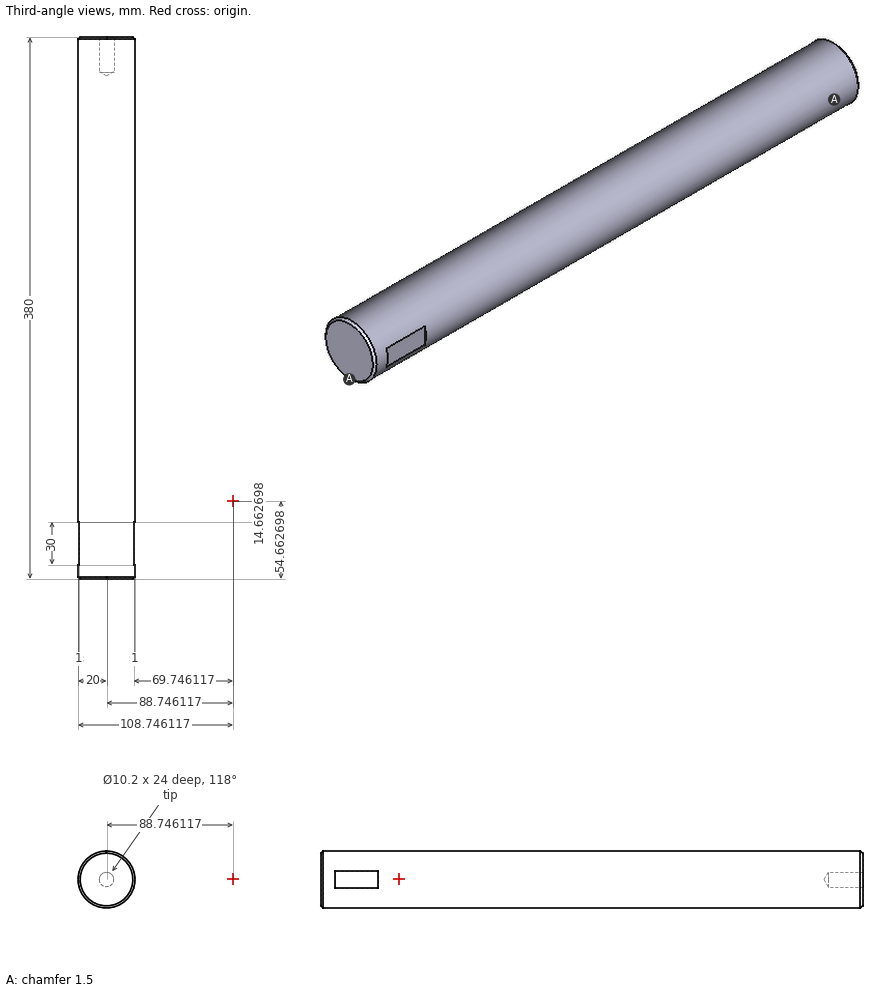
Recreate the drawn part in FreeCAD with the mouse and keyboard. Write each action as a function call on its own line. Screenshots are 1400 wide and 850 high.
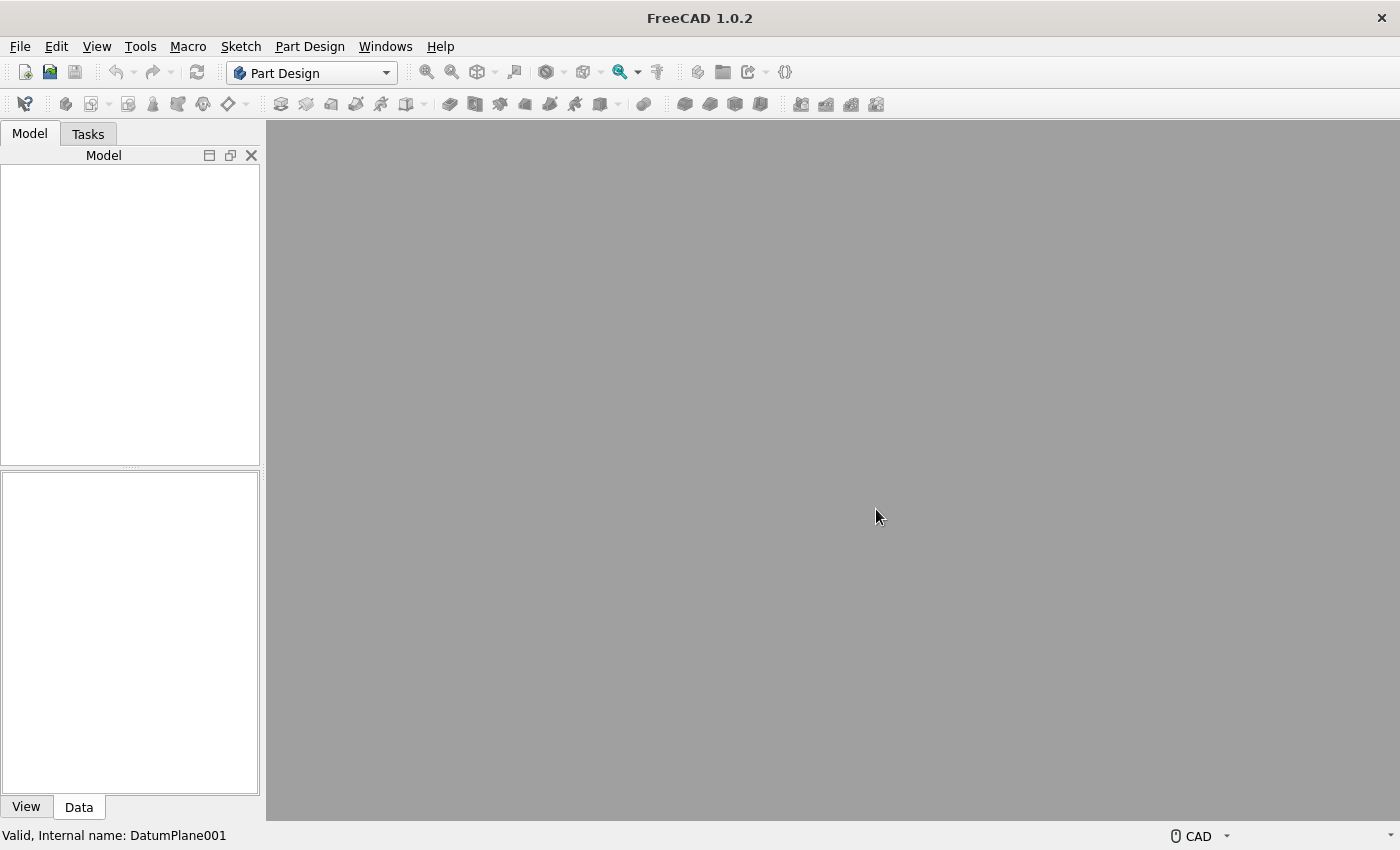
click(25, 72)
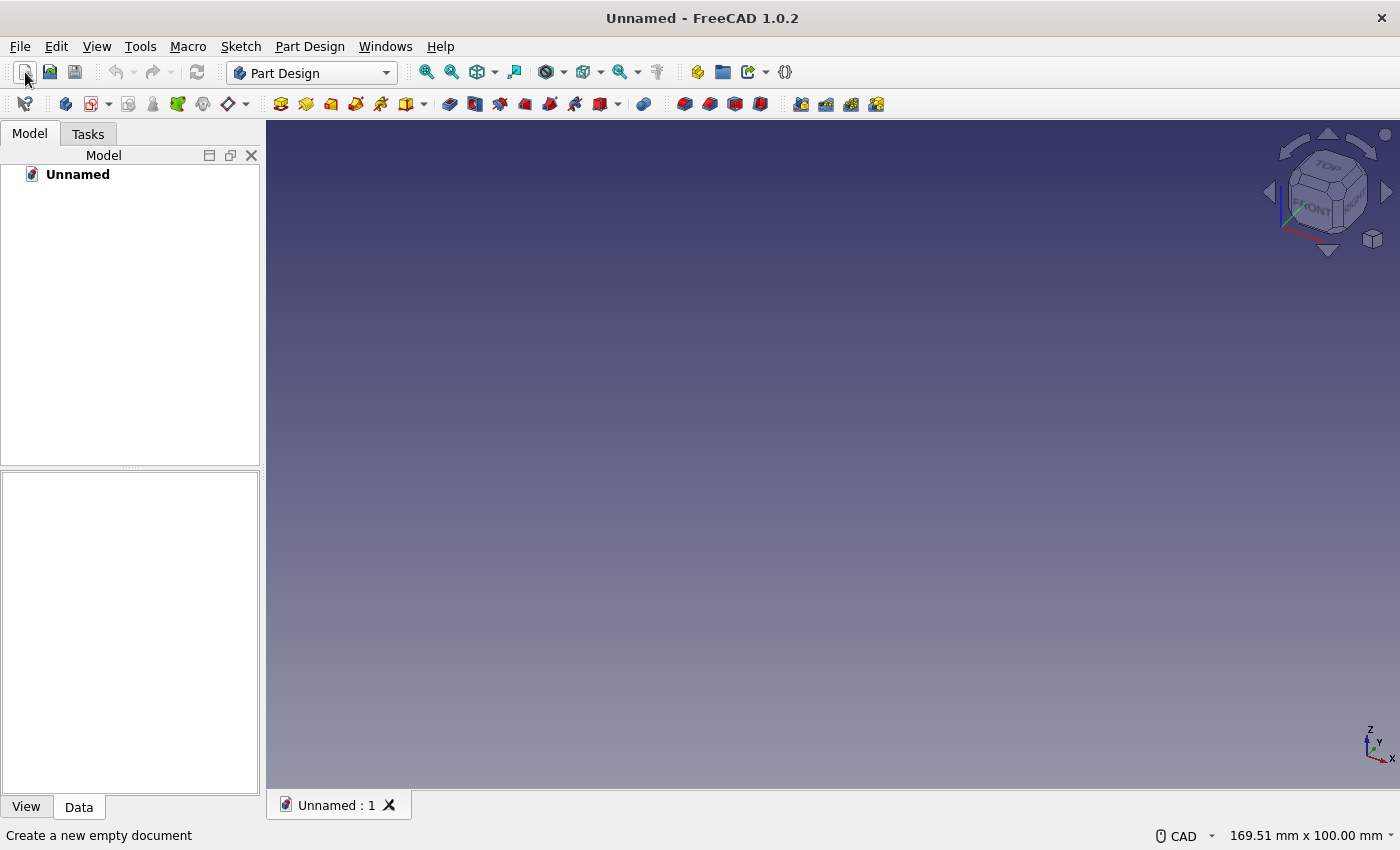
click(90, 104)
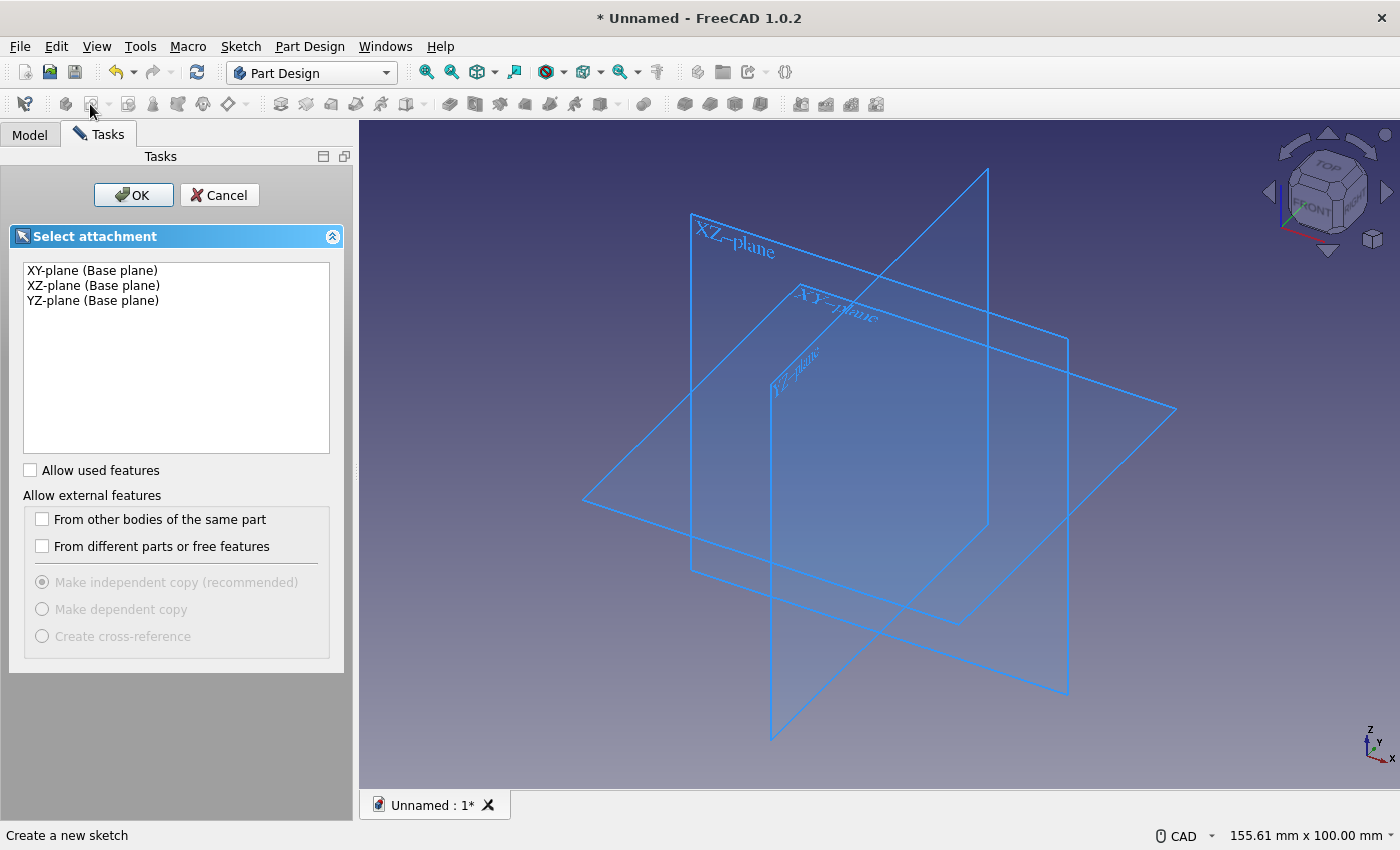
click(84, 270)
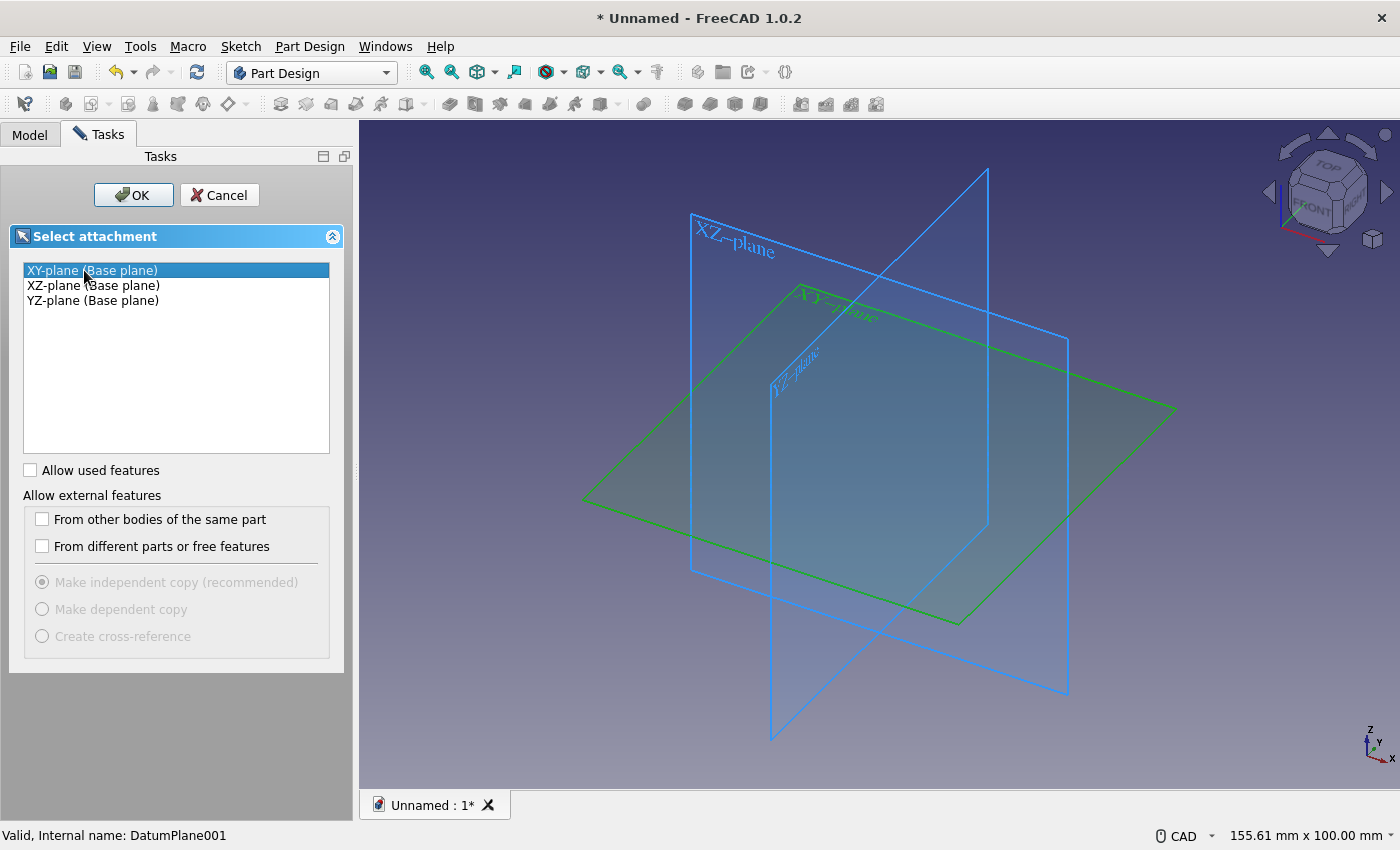
click(134, 195)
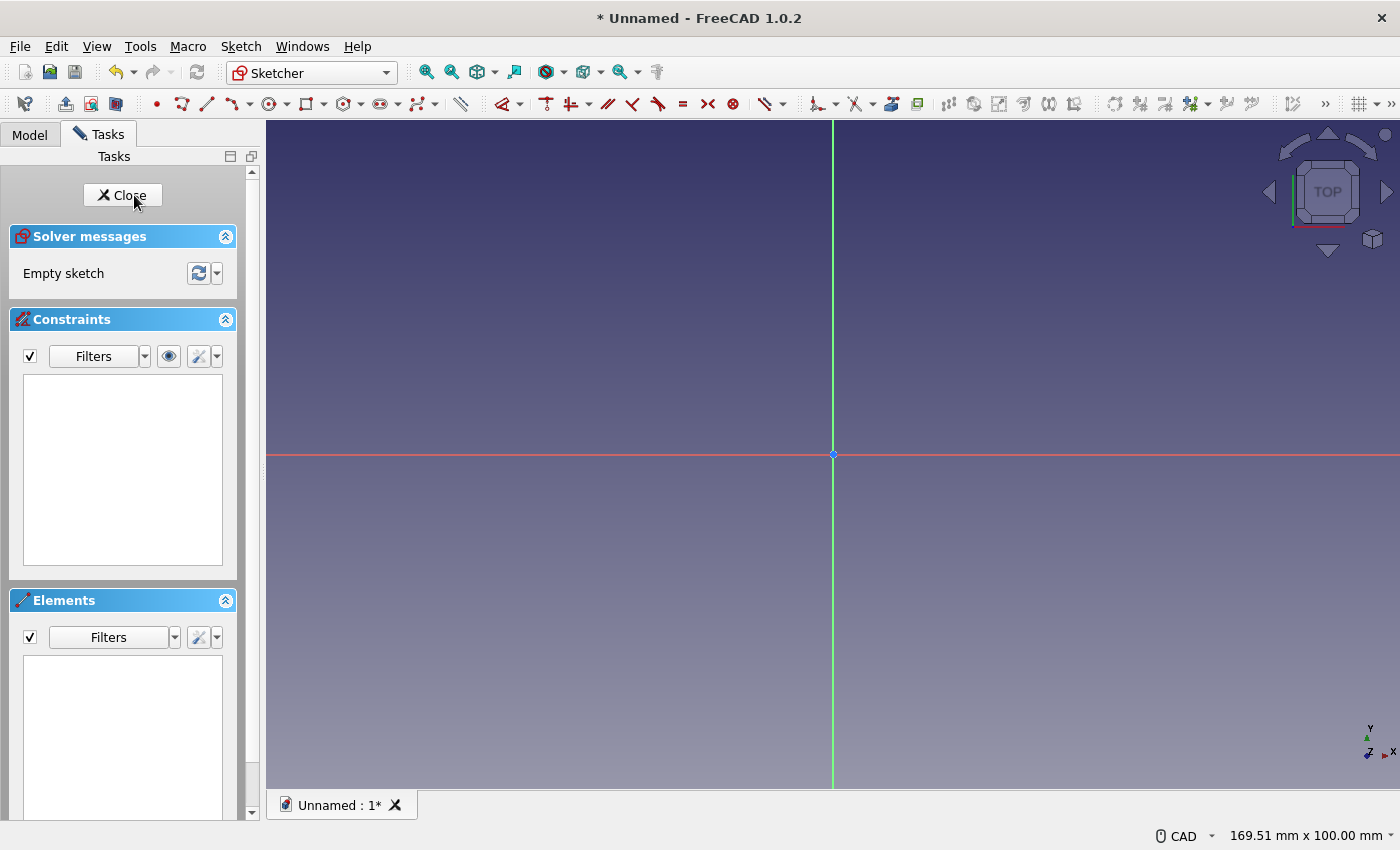
scroll(801, 504, down, 11)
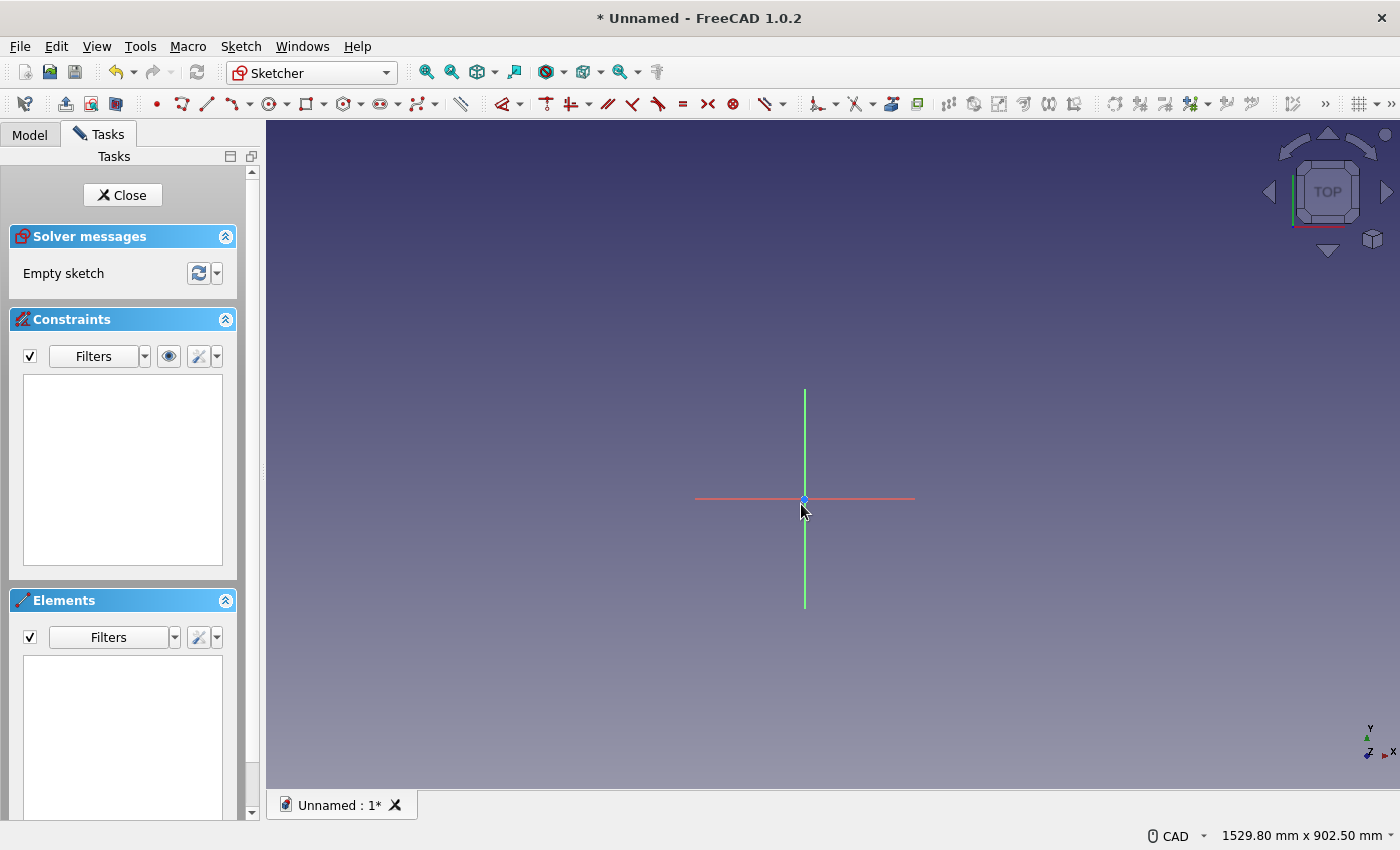
click(306, 104)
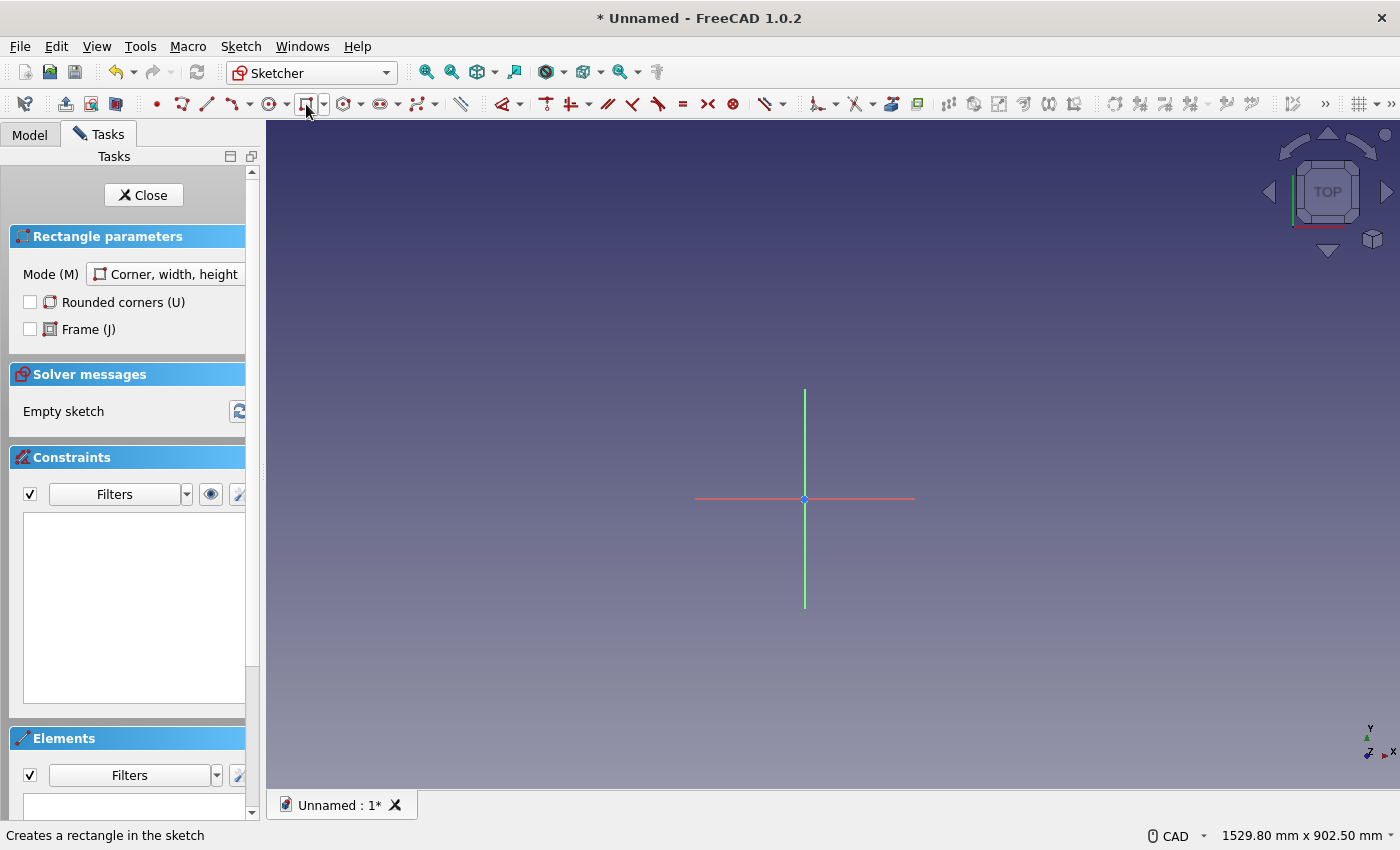
click(724, 258)
move(739, 540)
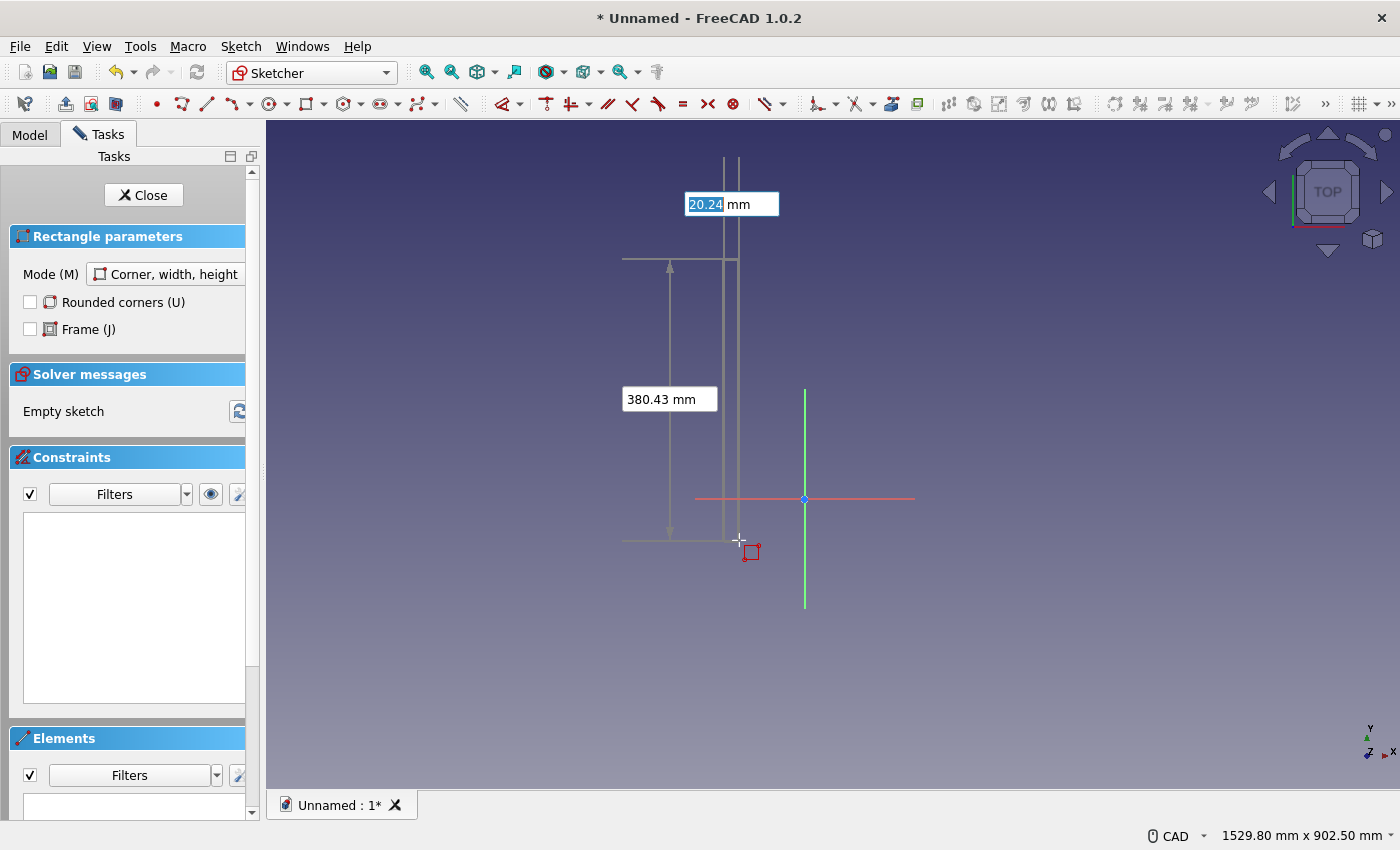
text(20)
key(Tab)
text(380)
key(Return)